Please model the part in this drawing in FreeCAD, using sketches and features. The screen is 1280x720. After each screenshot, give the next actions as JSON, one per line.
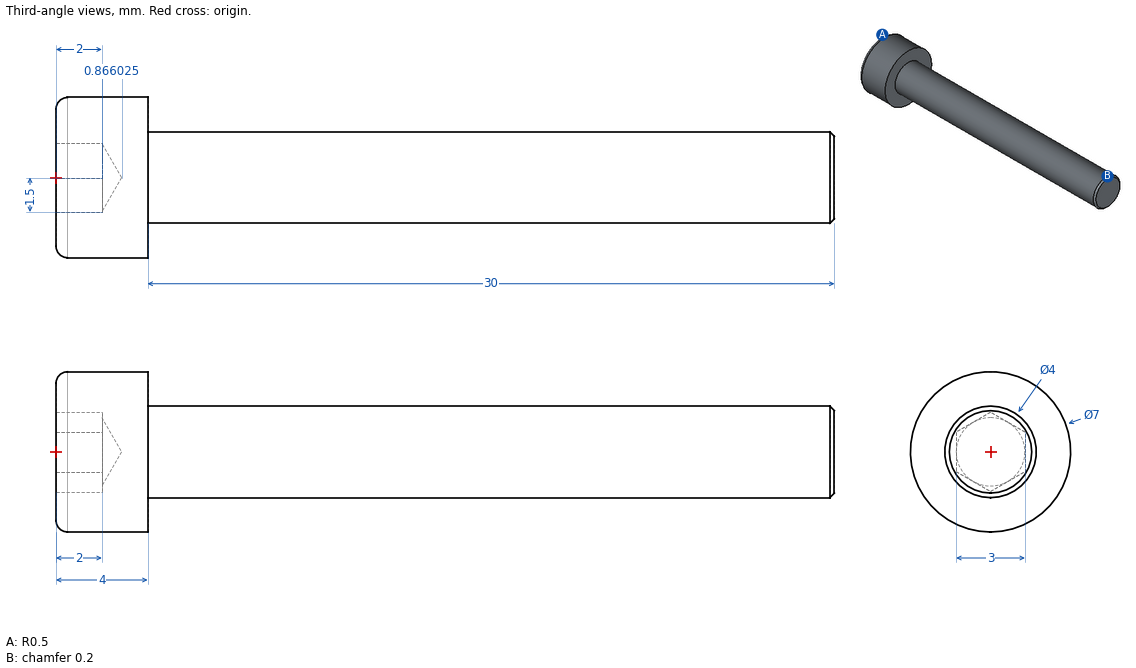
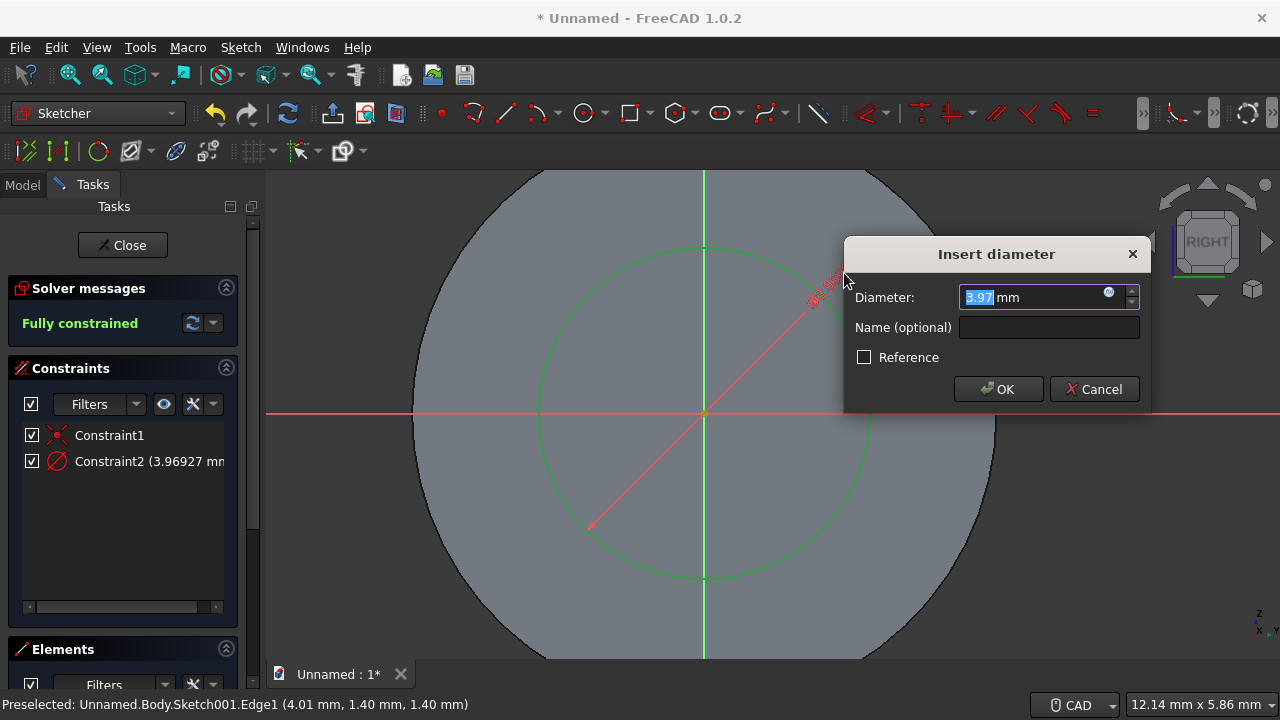
{"action": "type", "text": "4"}
{"action": "key", "text": "Return"}
{"action": "key", "text": "Escape"}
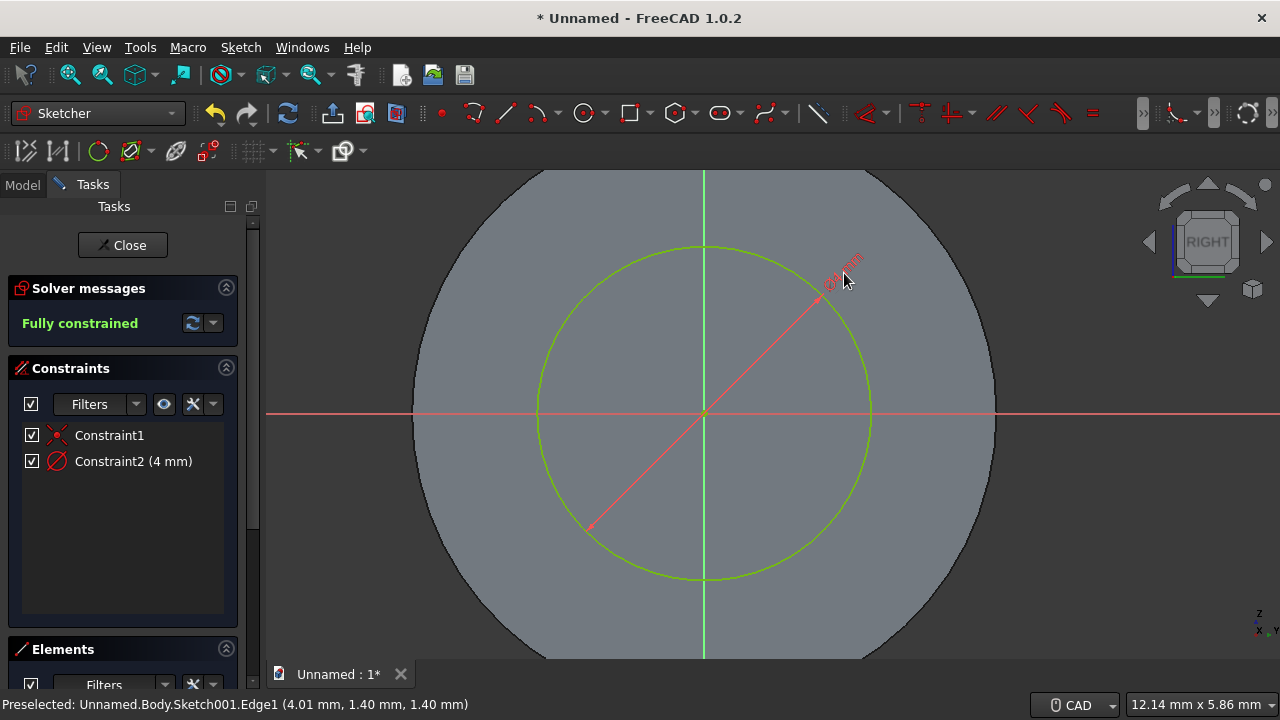
{"action": "left_click", "coordinate": [123, 245]}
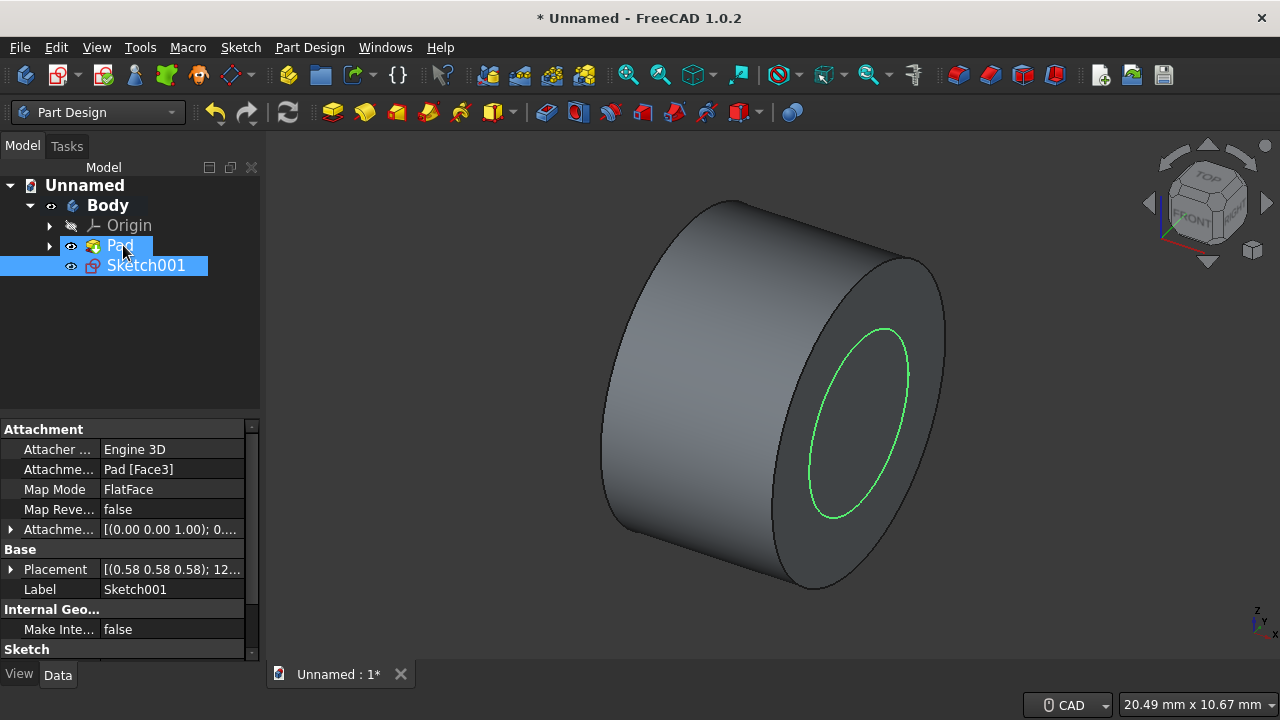
{"action": "left_click", "coordinate": [334, 112]}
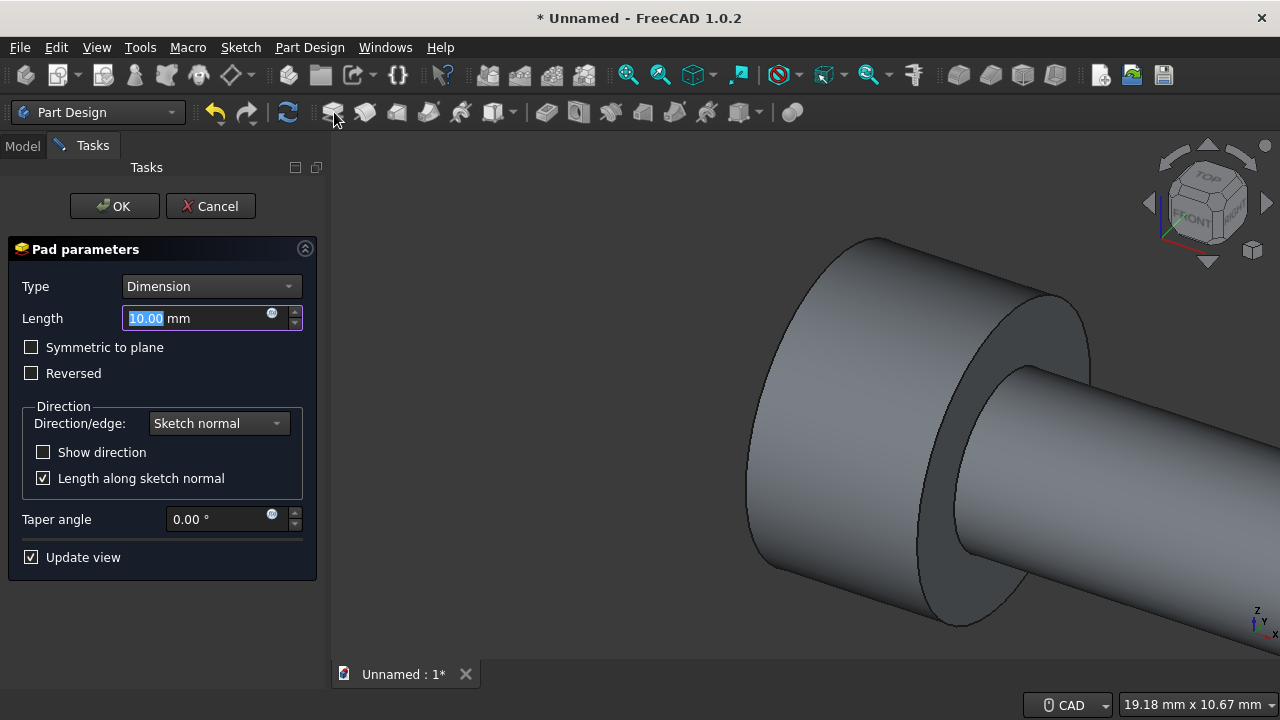
{"action": "type", "text": "30"}
{"action": "key", "text": "Tab"}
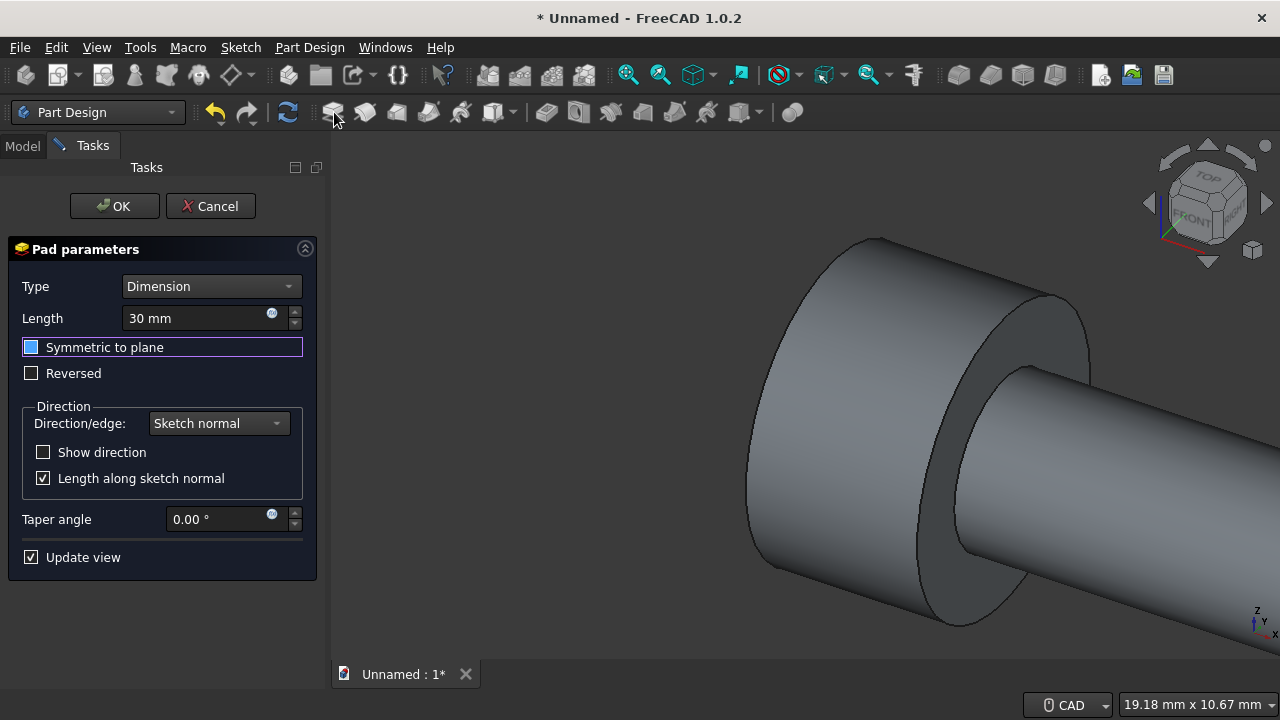
{"action": "left_click", "coordinate": [115, 206]}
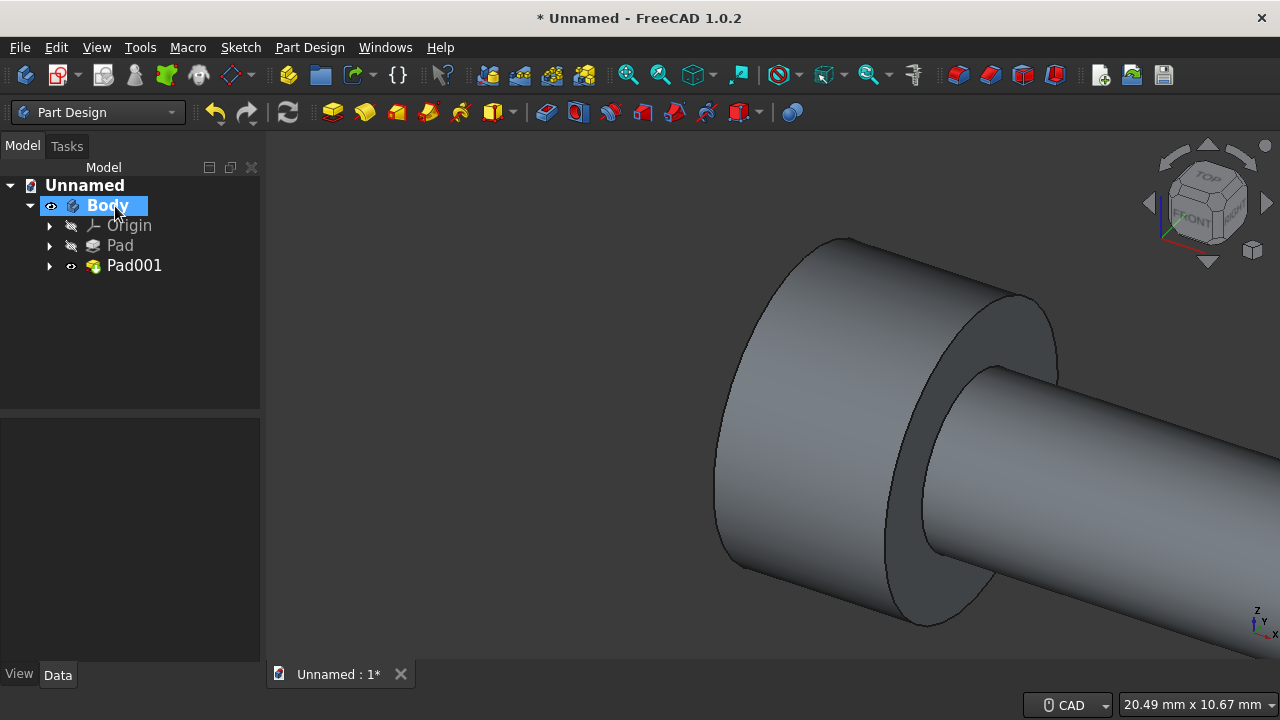
{"action": "left_click", "coordinate": [630, 76]}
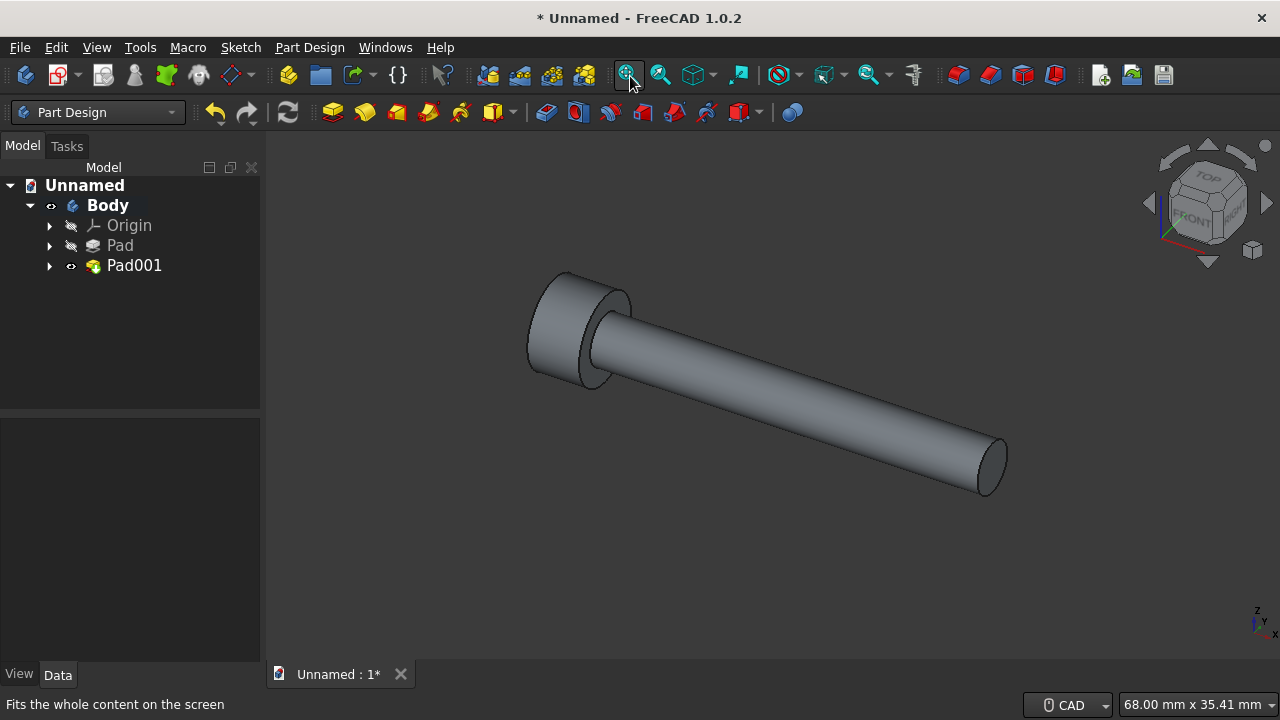
{"action": "key", "text": "6"}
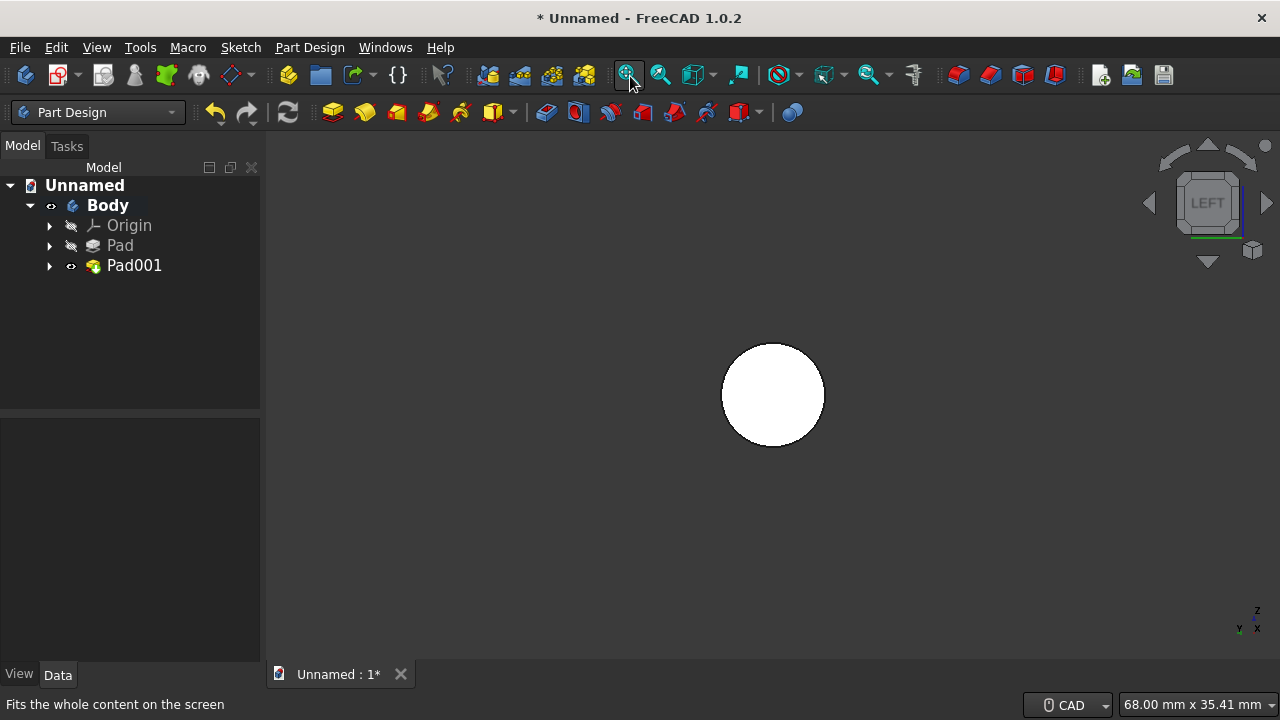
{"action": "left_click", "coordinate": [630, 76]}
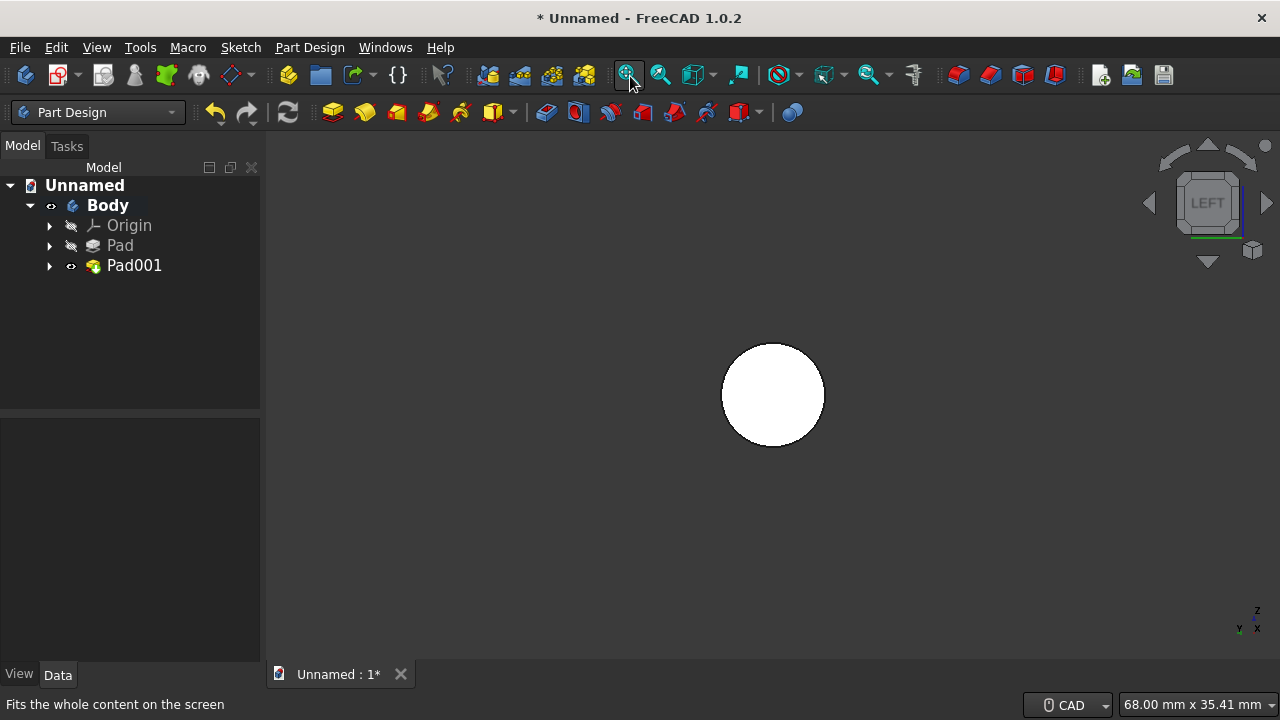
{"action": "left_click", "coordinate": [773, 394]}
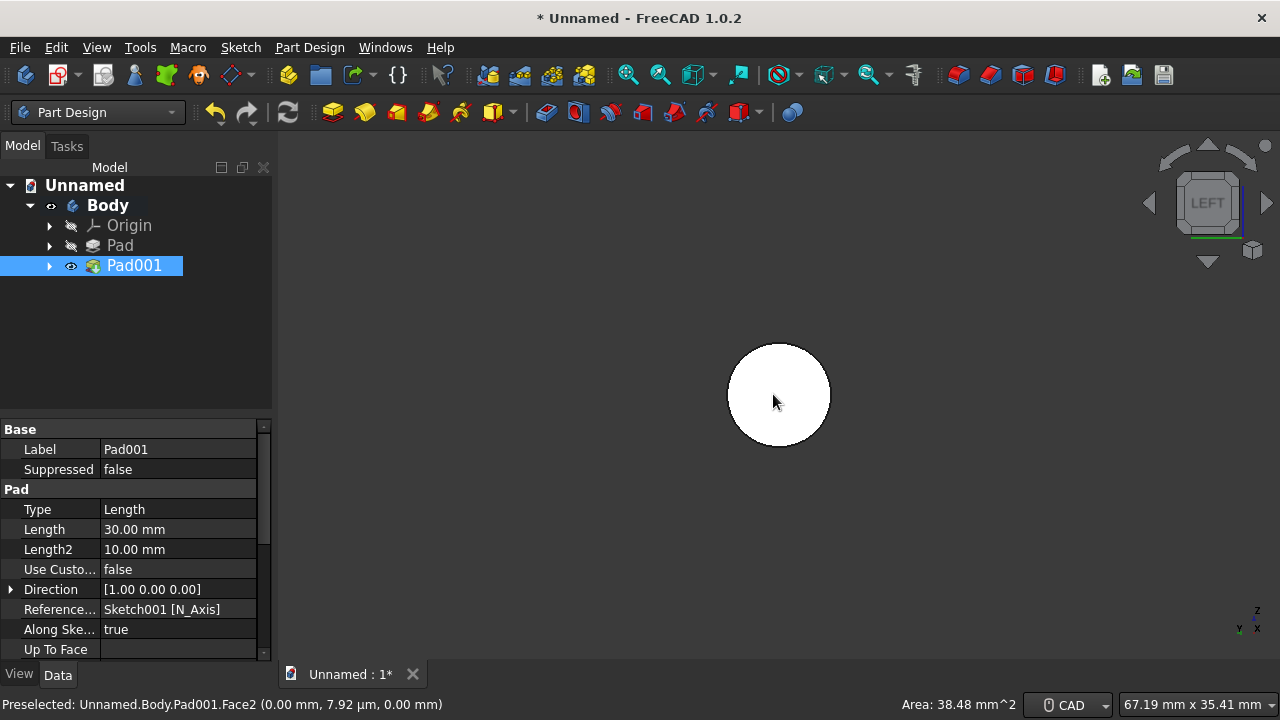
{"action": "left_click", "coordinate": [58, 76]}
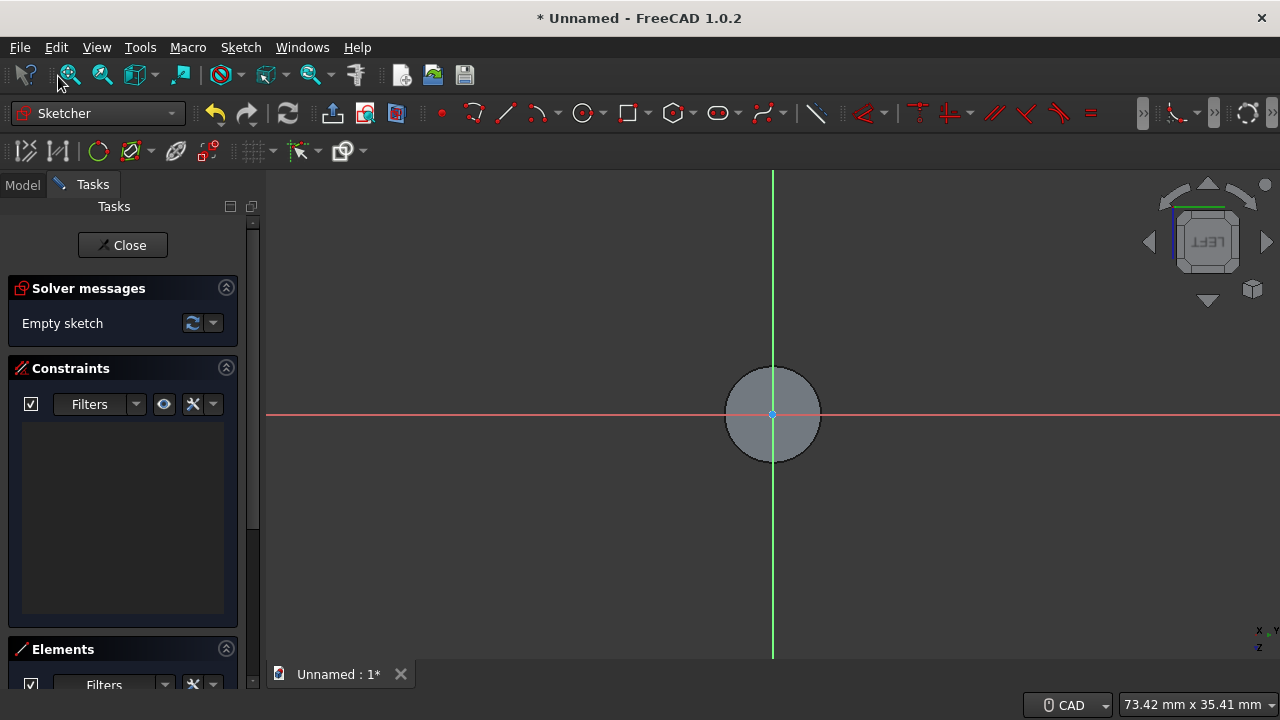
{"action": "scroll", "coordinate": [786, 414], "scroll_direction": "up", "scroll_amount": 9}